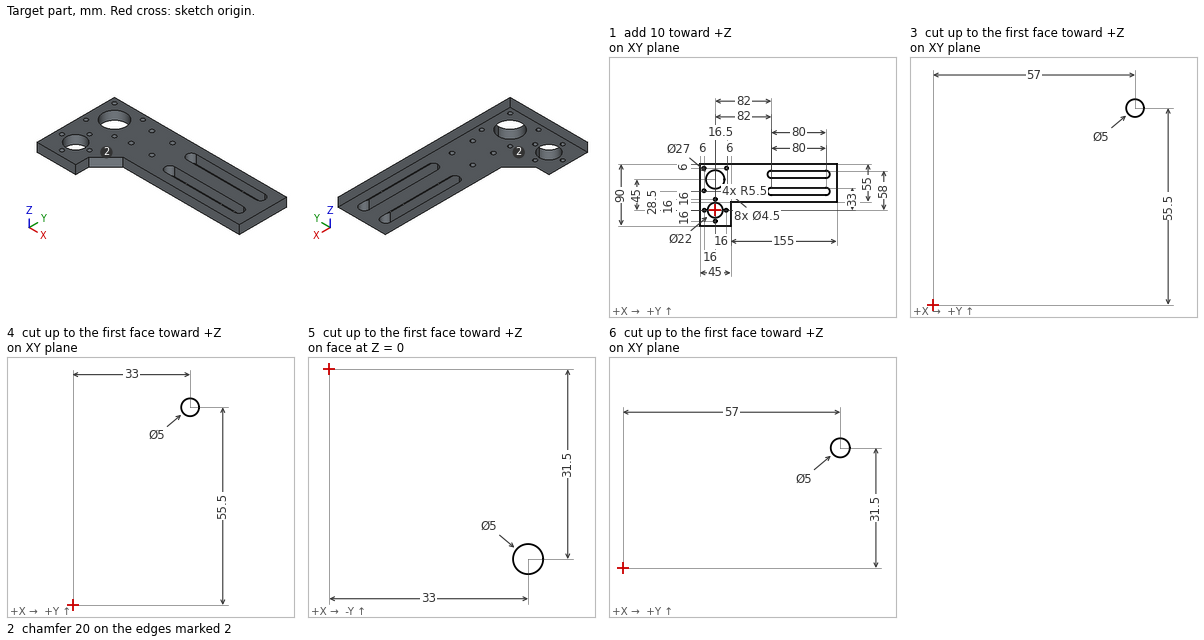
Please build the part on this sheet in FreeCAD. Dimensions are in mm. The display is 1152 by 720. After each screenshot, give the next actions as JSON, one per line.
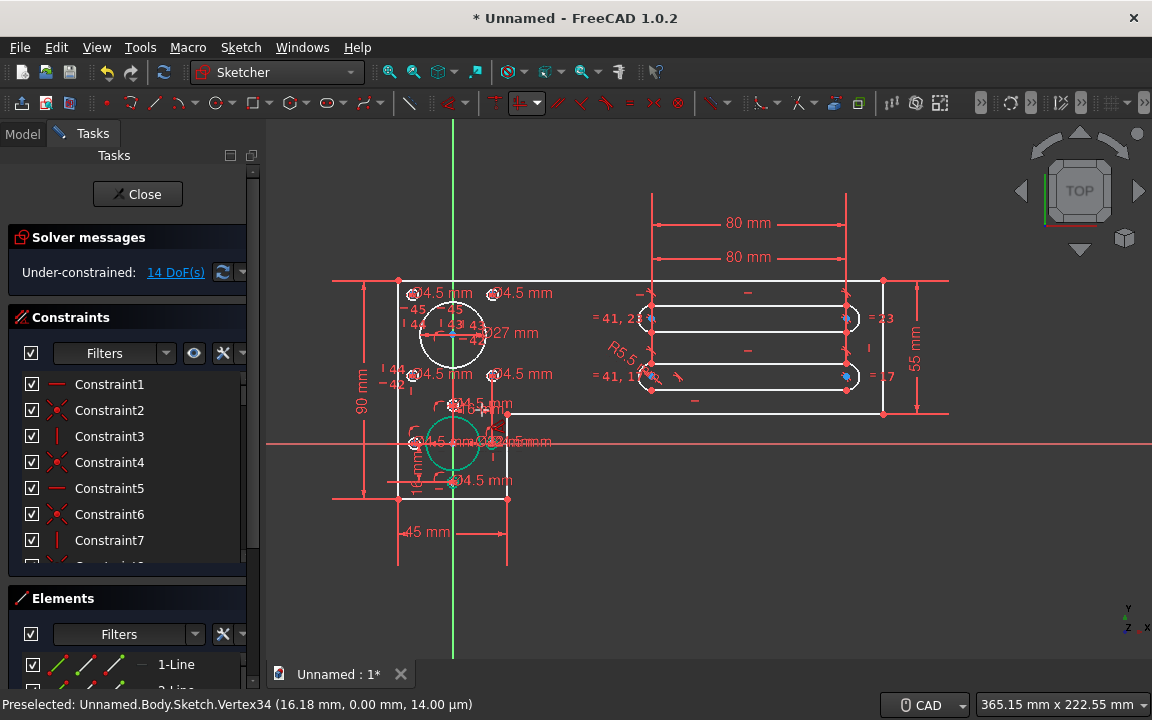
{"action": "left_click", "coordinate": [414, 444]}
{"action": "left_click", "coordinate": [434, 338]}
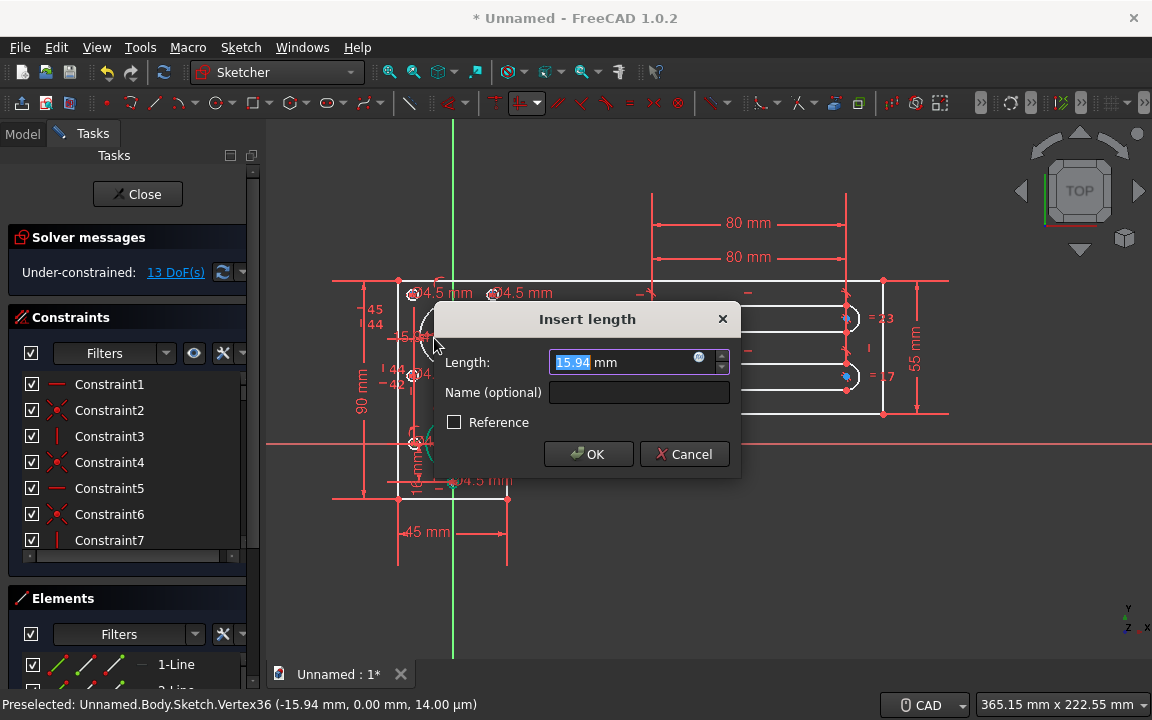
{"action": "type", "text": "16"}
{"action": "key", "text": "Return"}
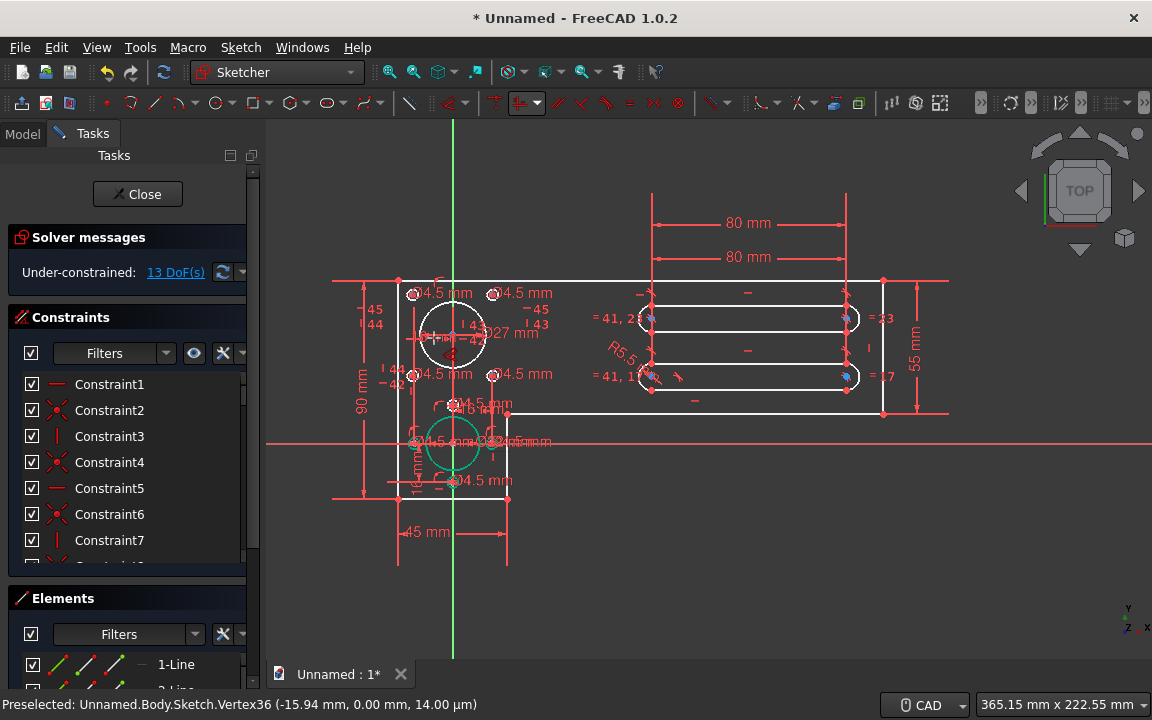
{"action": "left_click", "coordinate": [453, 406]}
{"action": "left_click", "coordinate": [371, 425]}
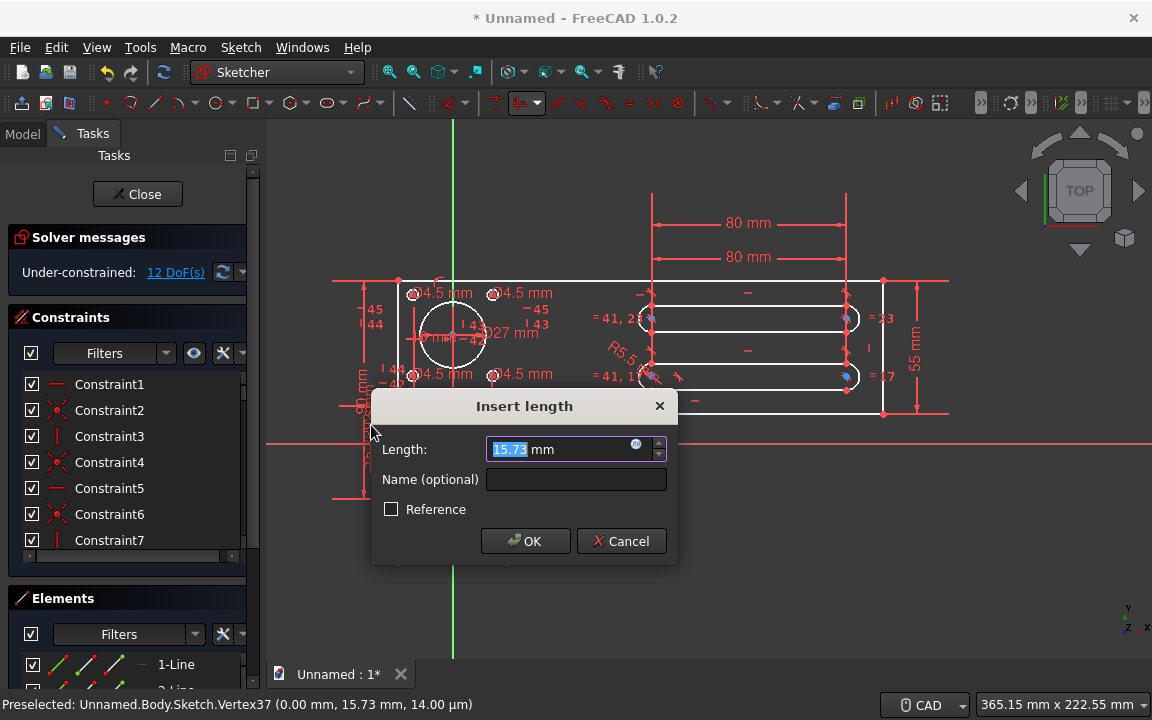
{"action": "type", "text": "16"}
{"action": "key", "text": "Return"}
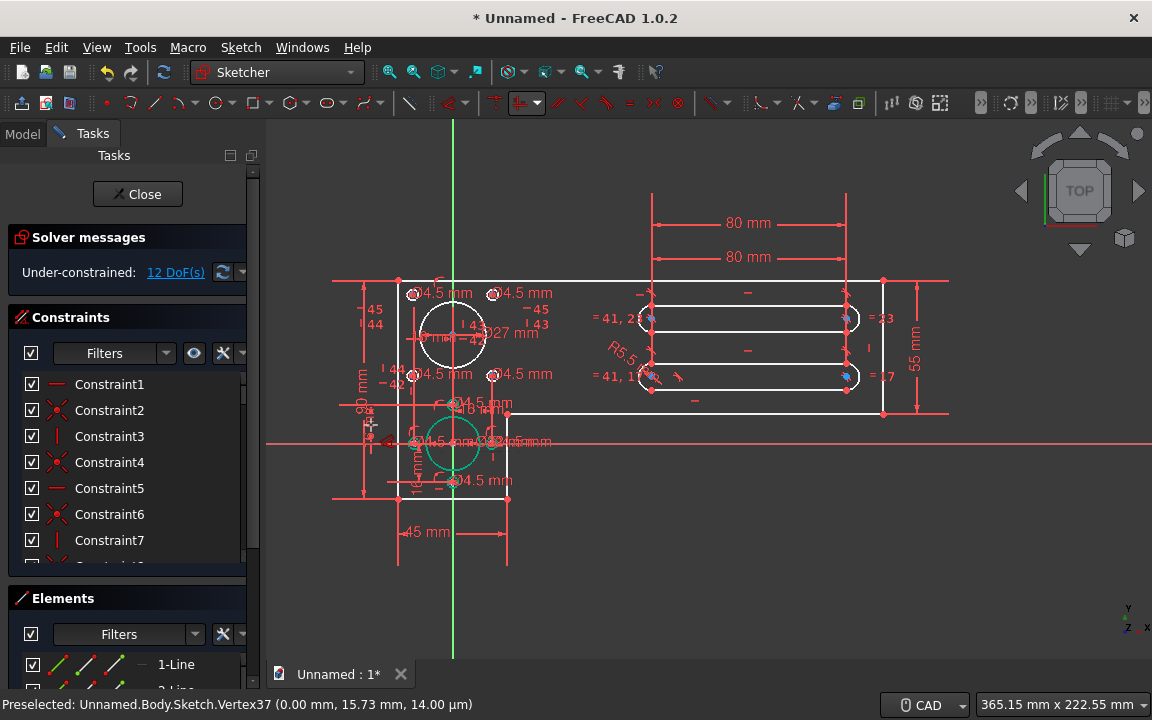
{"action": "left_click", "coordinate": [453, 335]}
{"action": "left_click", "coordinate": [511, 389]}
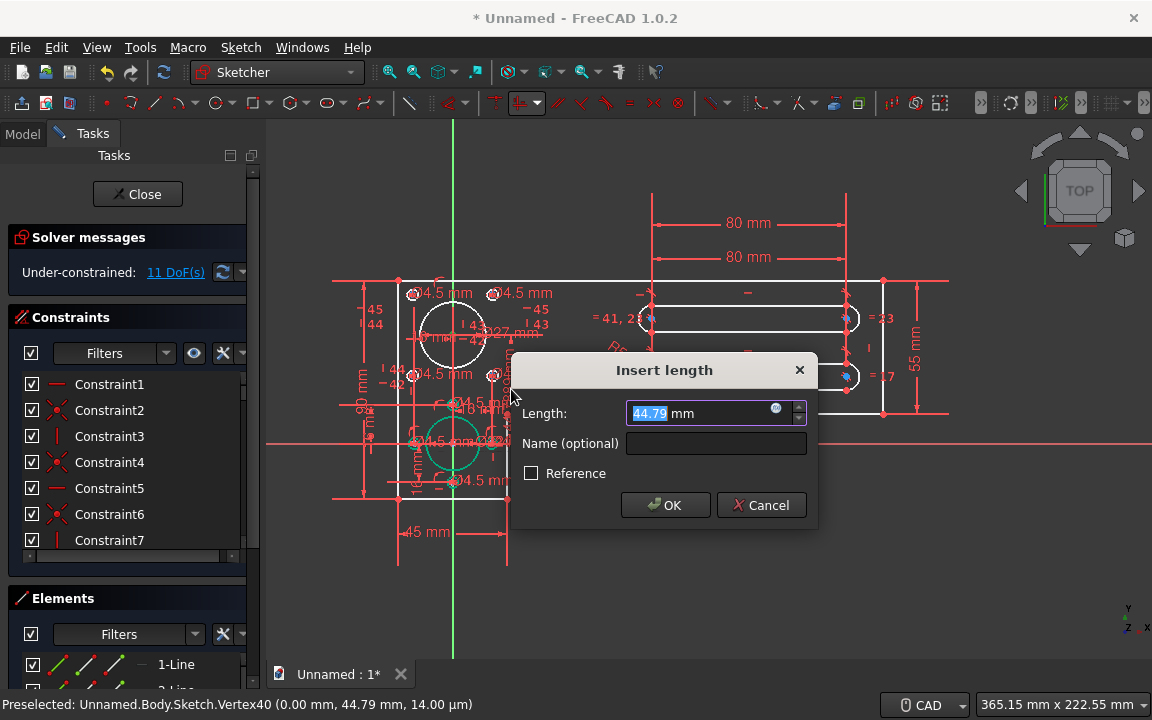
{"action": "type", "text": "45"}
{"action": "key", "text": "Return"}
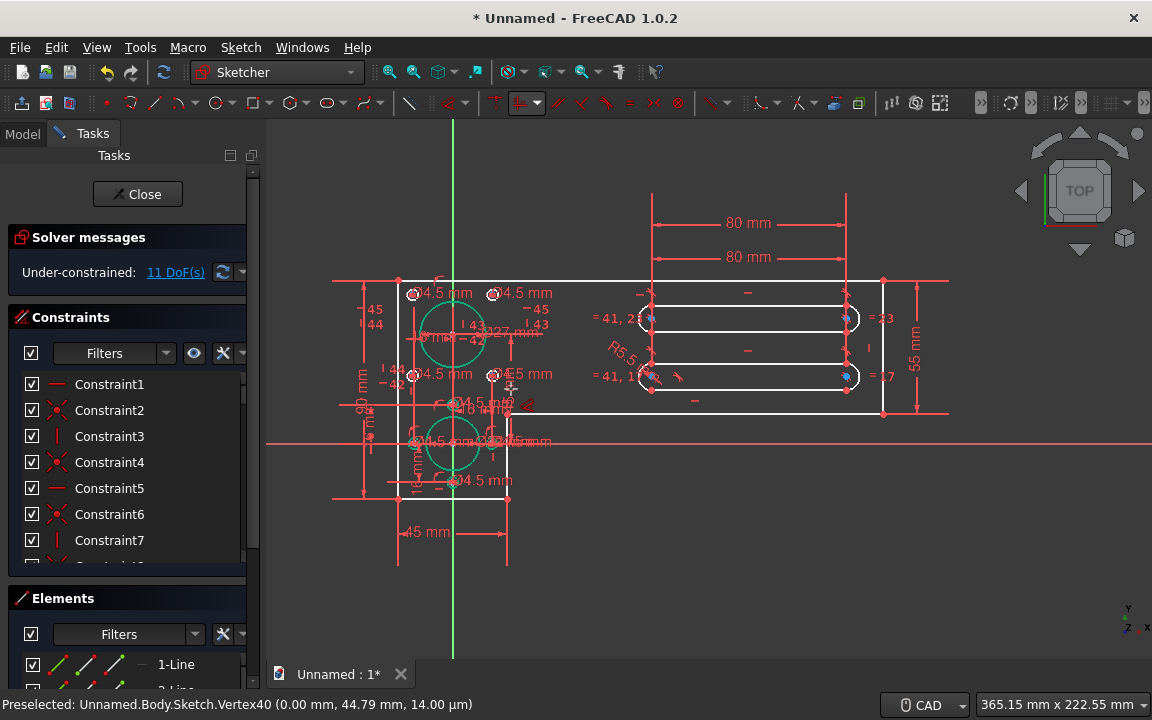
{"action": "scroll", "coordinate": [507, 414], "scroll_direction": "up", "scroll_amount": 6}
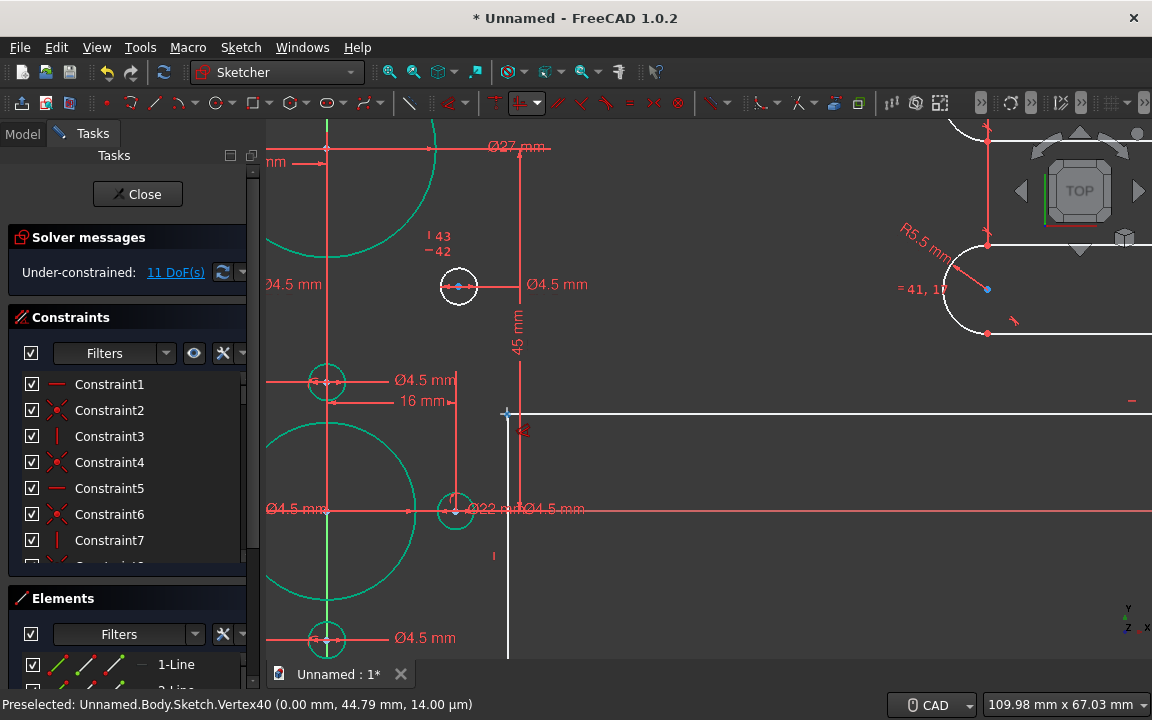
{"action": "left_click", "coordinate": [508, 414]}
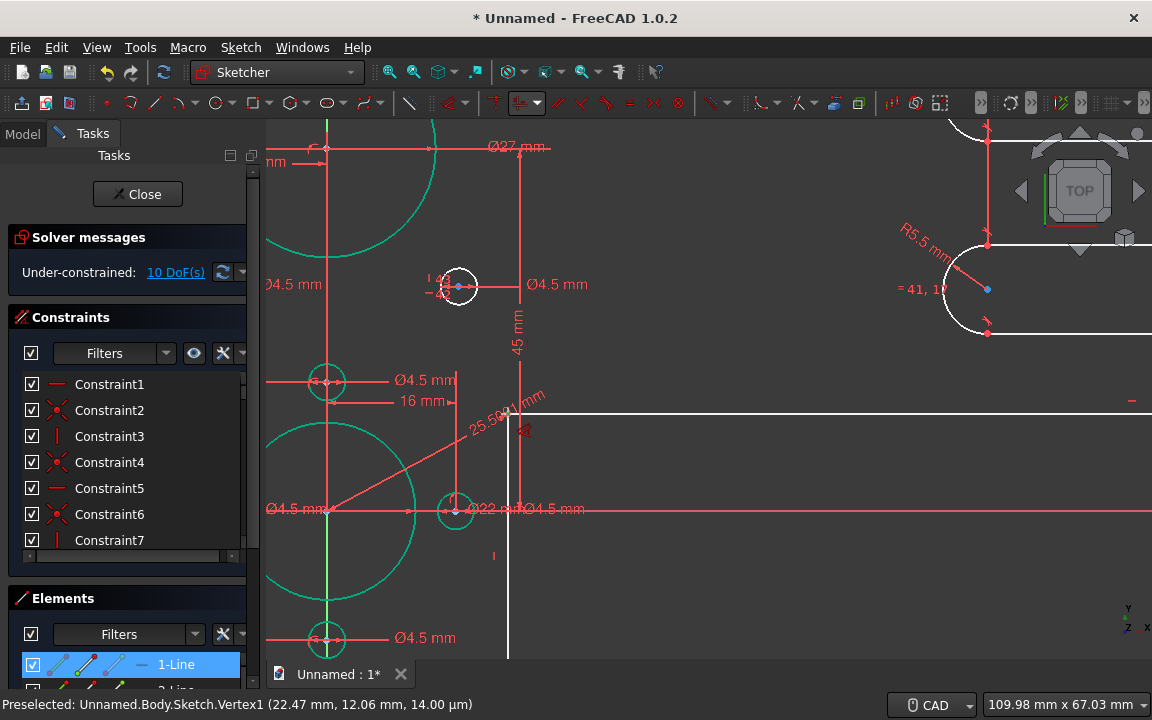
{"action": "left_click", "coordinate": [459, 287]}
{"action": "left_click", "coordinate": [483, 448]}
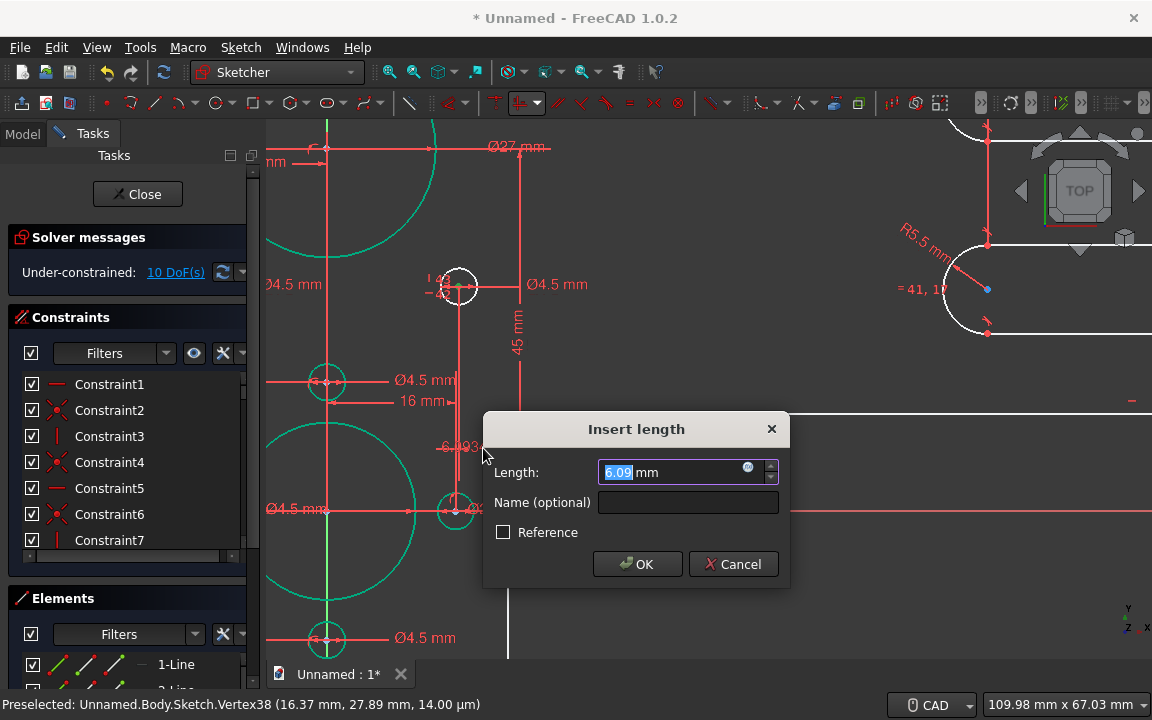
{"action": "type", "text": "6"}
{"action": "key", "text": "Return"}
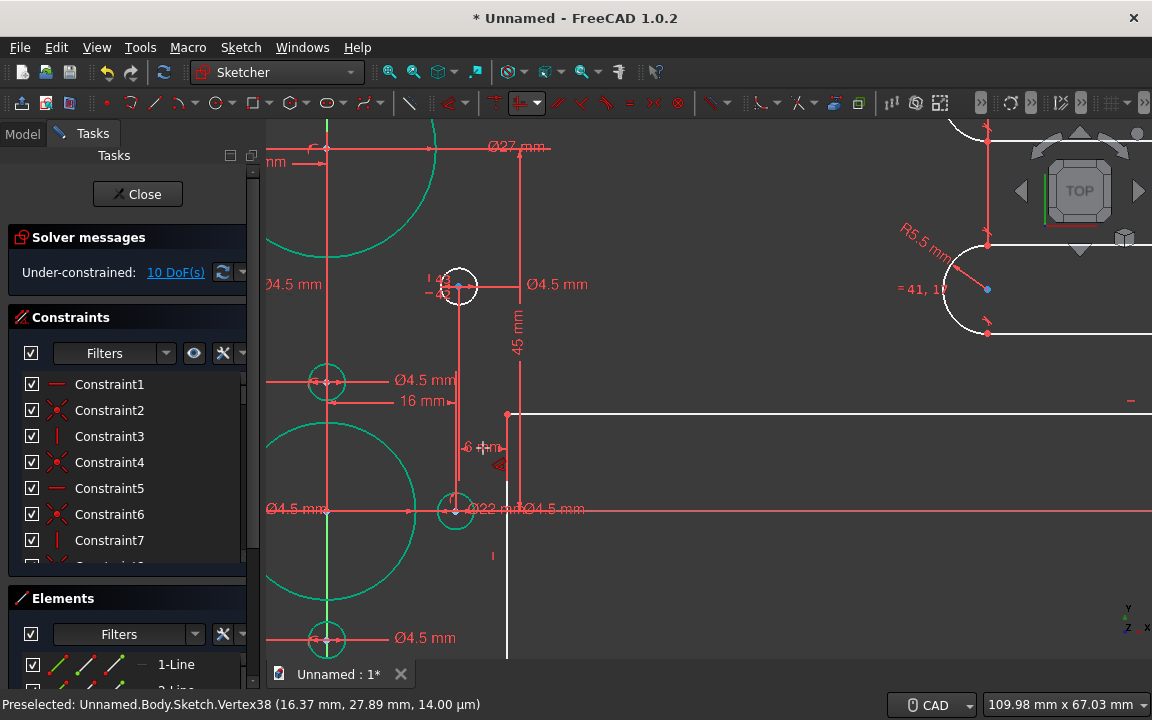
{"action": "scroll", "coordinate": [507, 414], "scroll_direction": "down", "scroll_amount": 6}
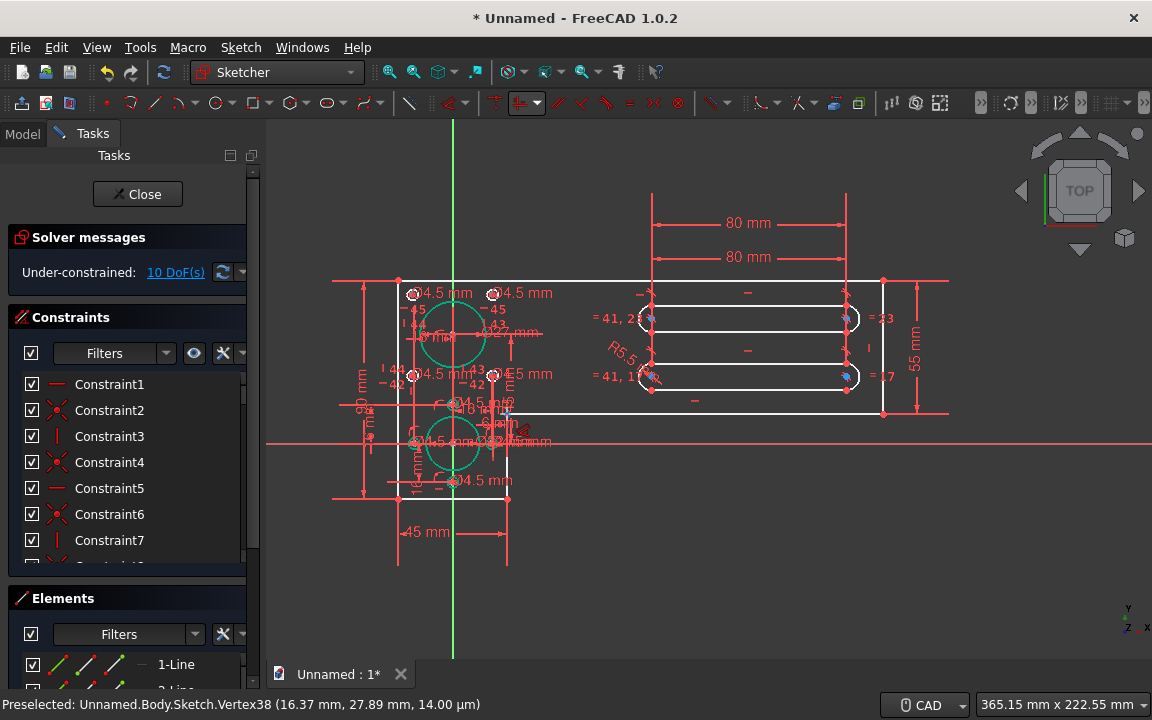
{"action": "scroll", "coordinate": [398, 281], "scroll_direction": "up", "scroll_amount": 6}